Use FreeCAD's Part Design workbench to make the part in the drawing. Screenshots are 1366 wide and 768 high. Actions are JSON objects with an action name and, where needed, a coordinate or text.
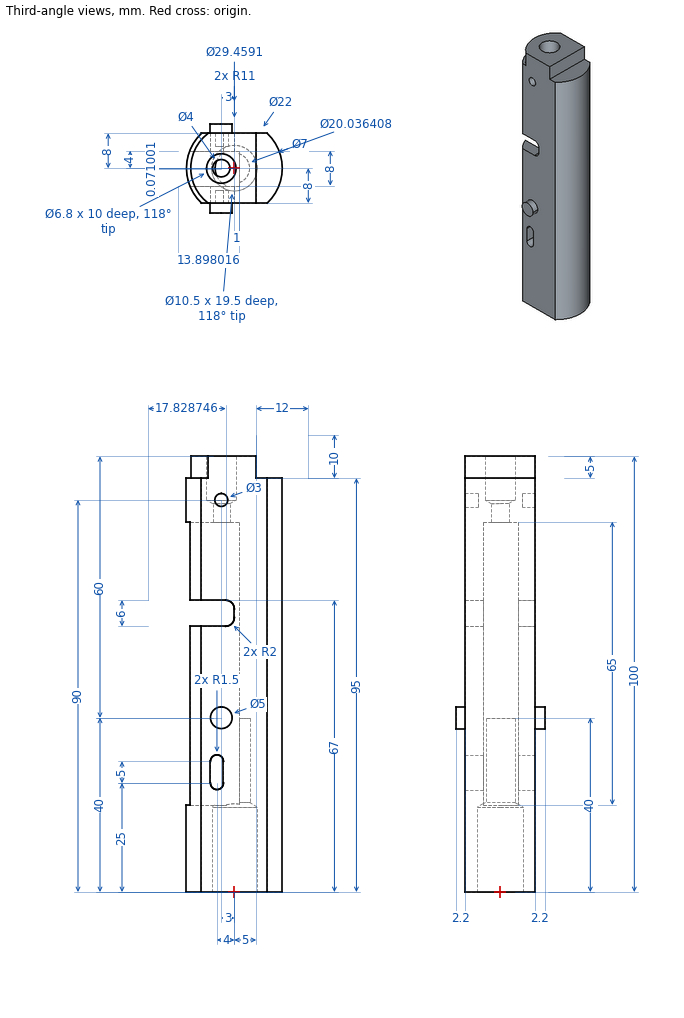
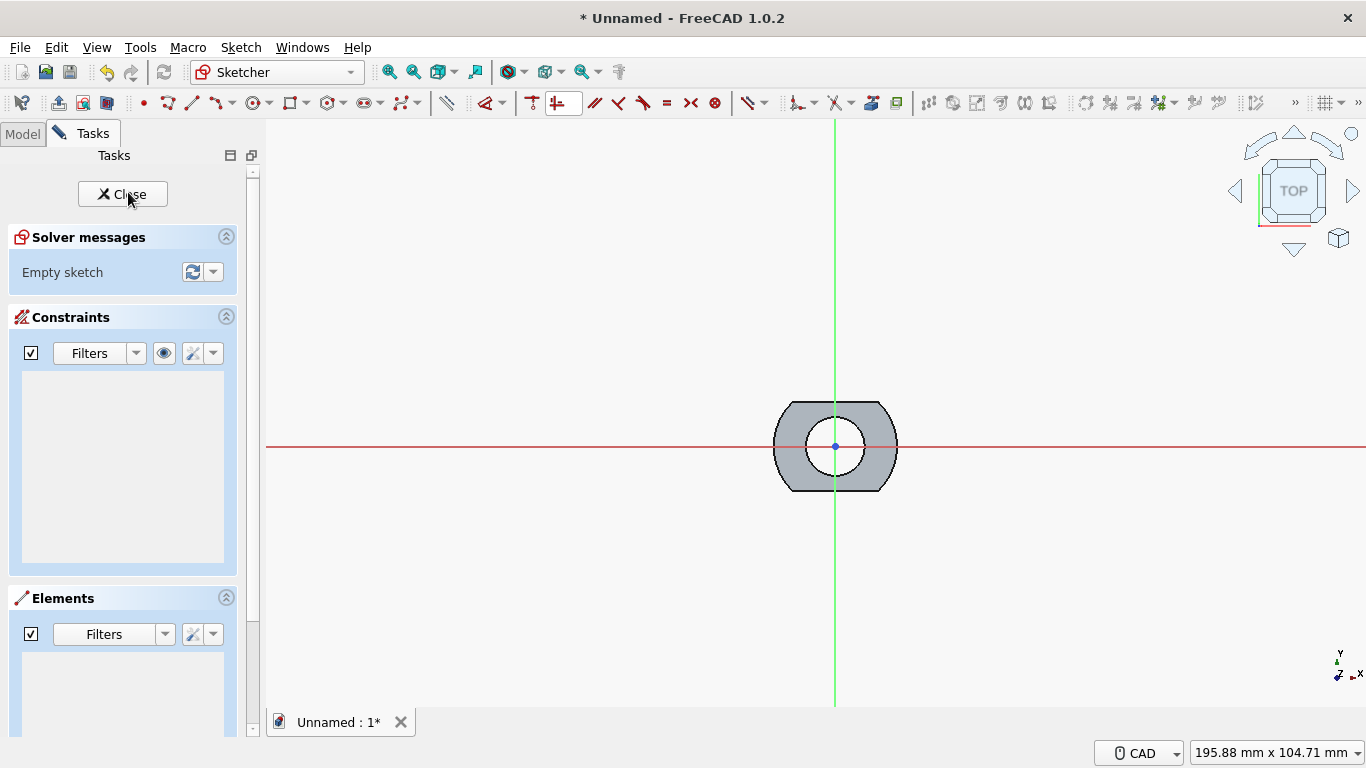
{"action": "scroll", "coordinate": [846, 451], "scroll_direction": "up", "scroll_amount": 11}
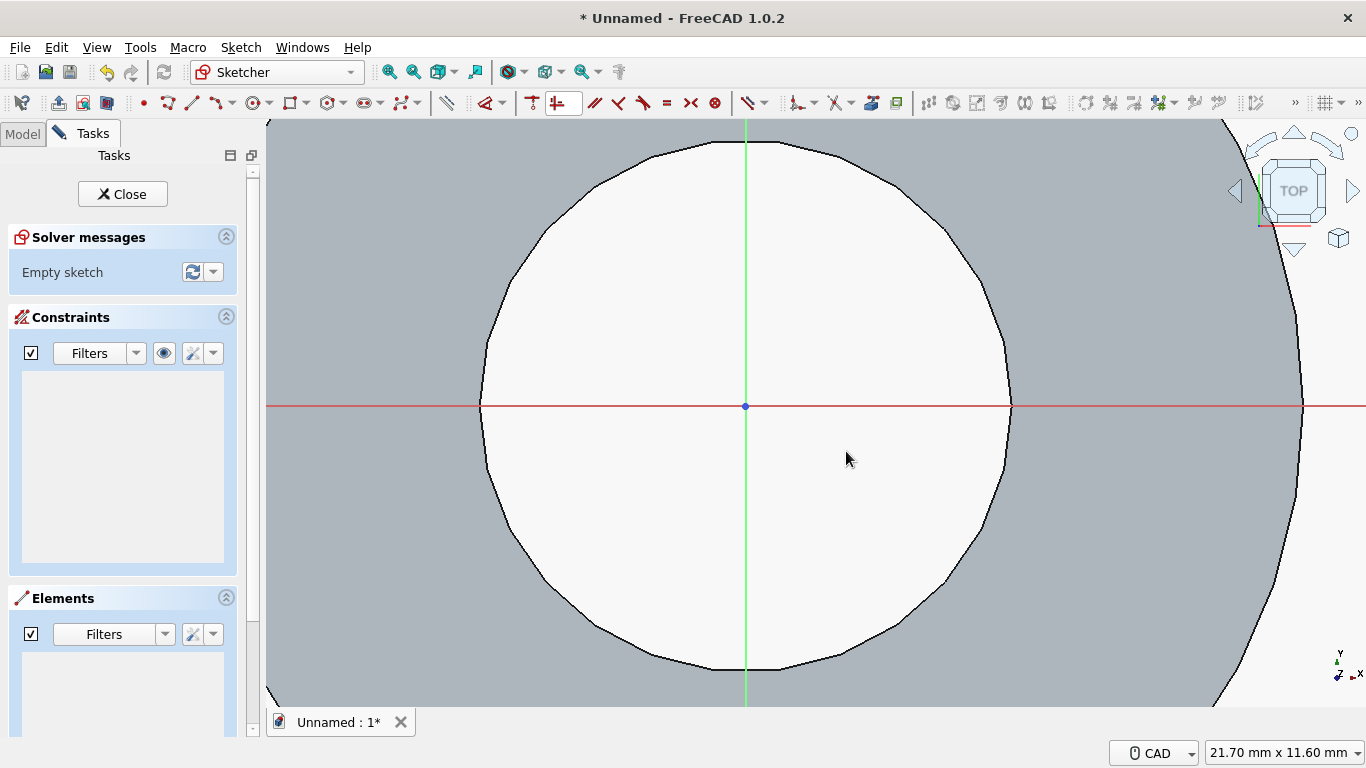
{"action": "left_click", "coordinate": [254, 104]}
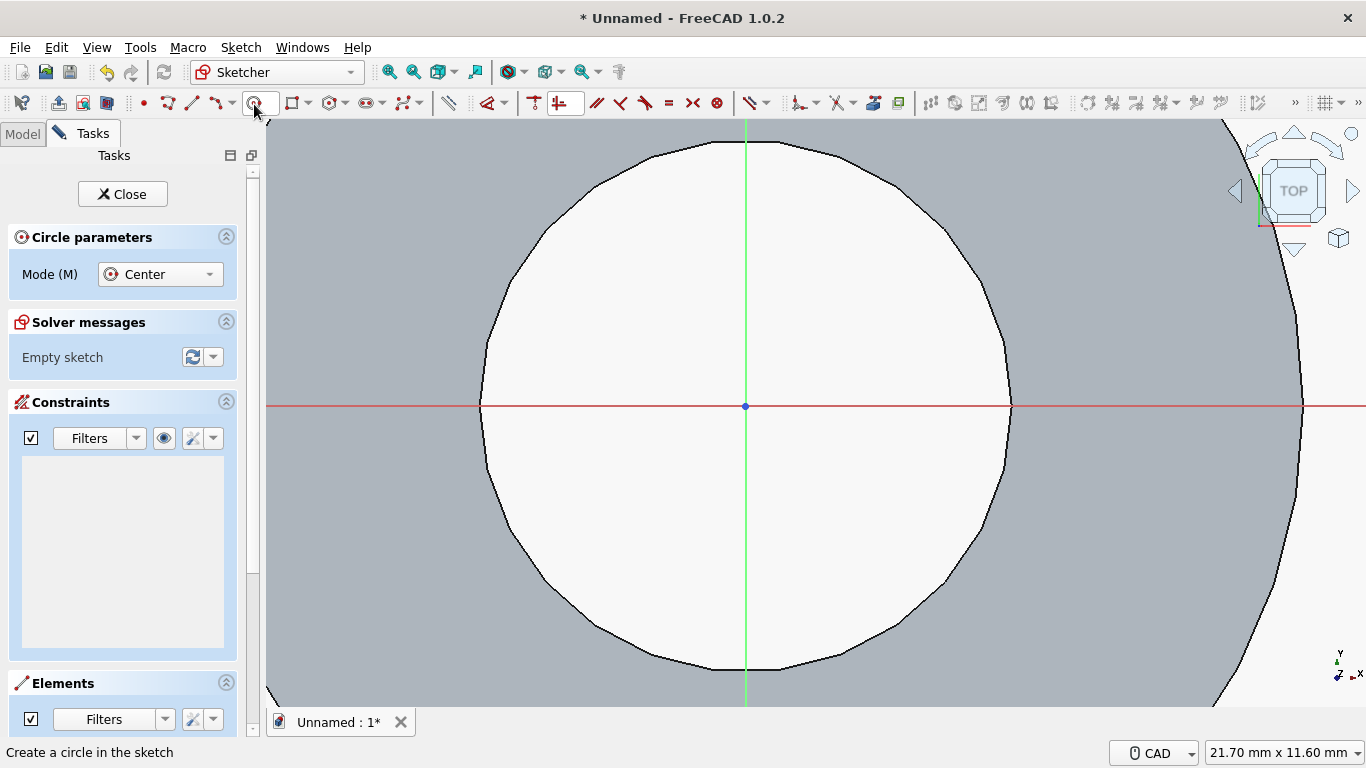
{"action": "left_click", "coordinate": [746, 406]}
{"action": "mouse_move", "coordinate": [871, 281]}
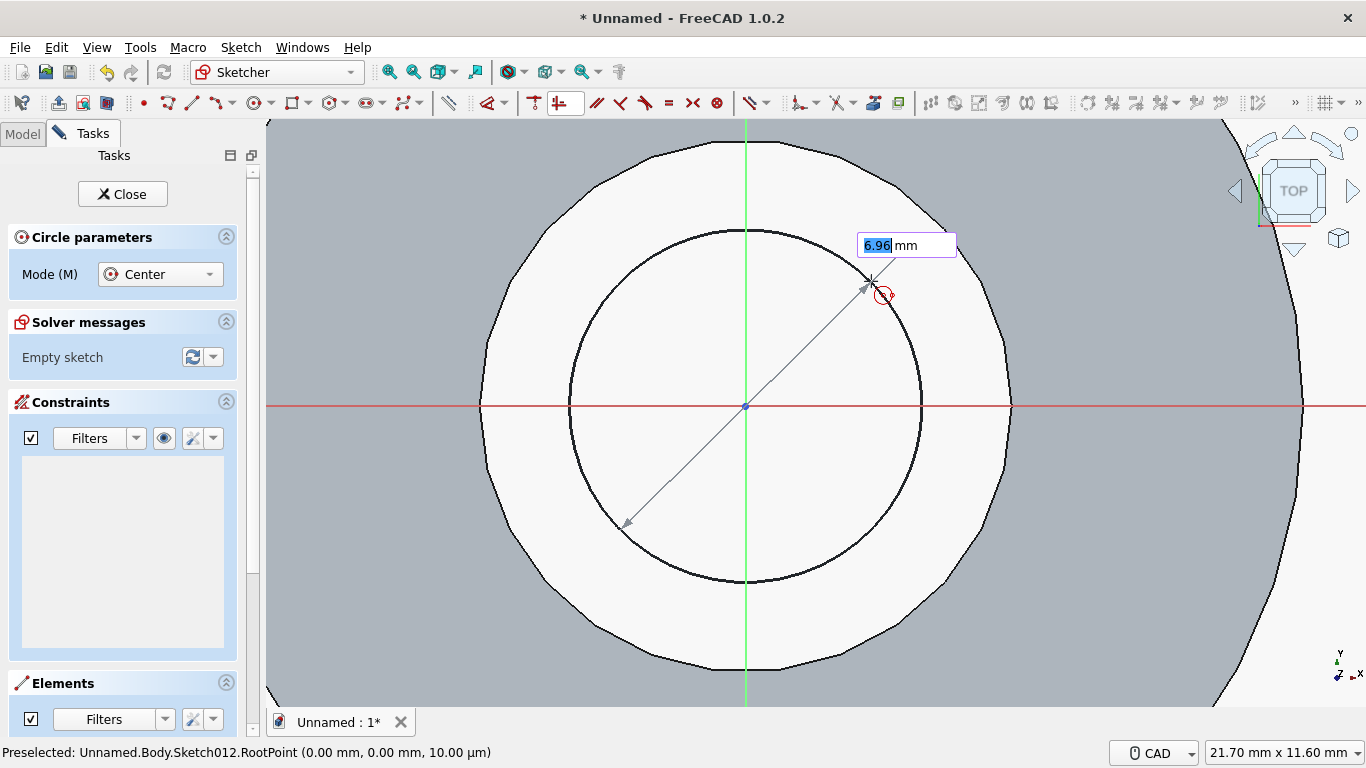
{"action": "type", "text": "7"}
{"action": "key", "text": "Return"}
{"action": "key", "text": "Escape"}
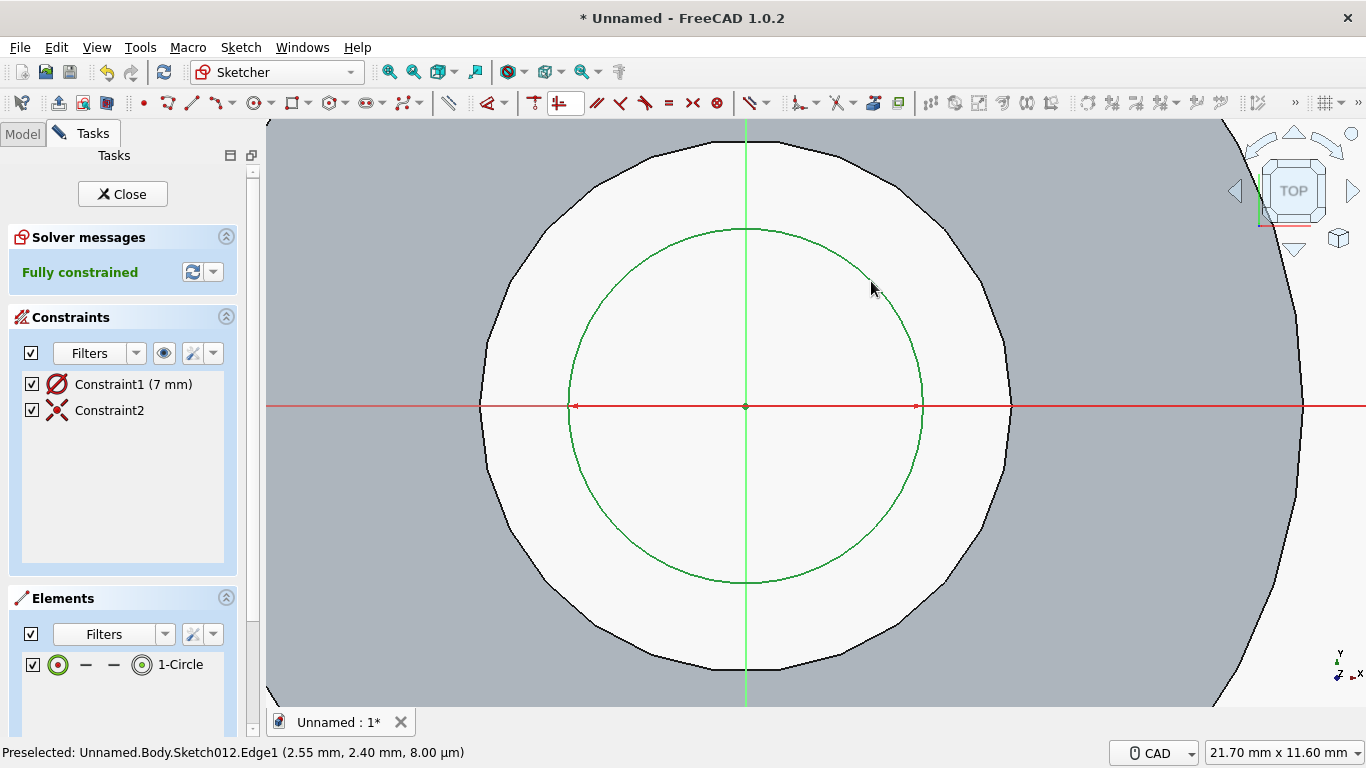
{"action": "left_click", "coordinate": [123, 194]}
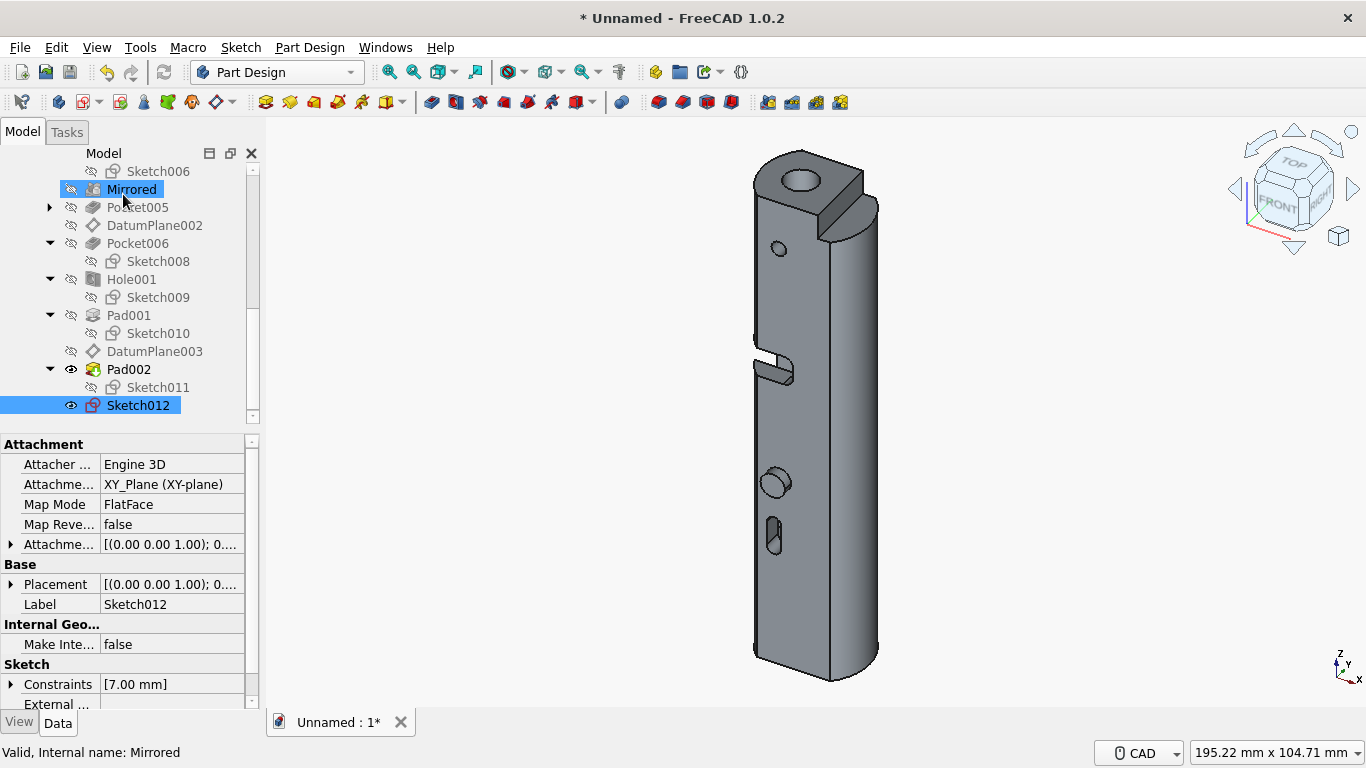
{"action": "left_click", "coordinate": [432, 102]}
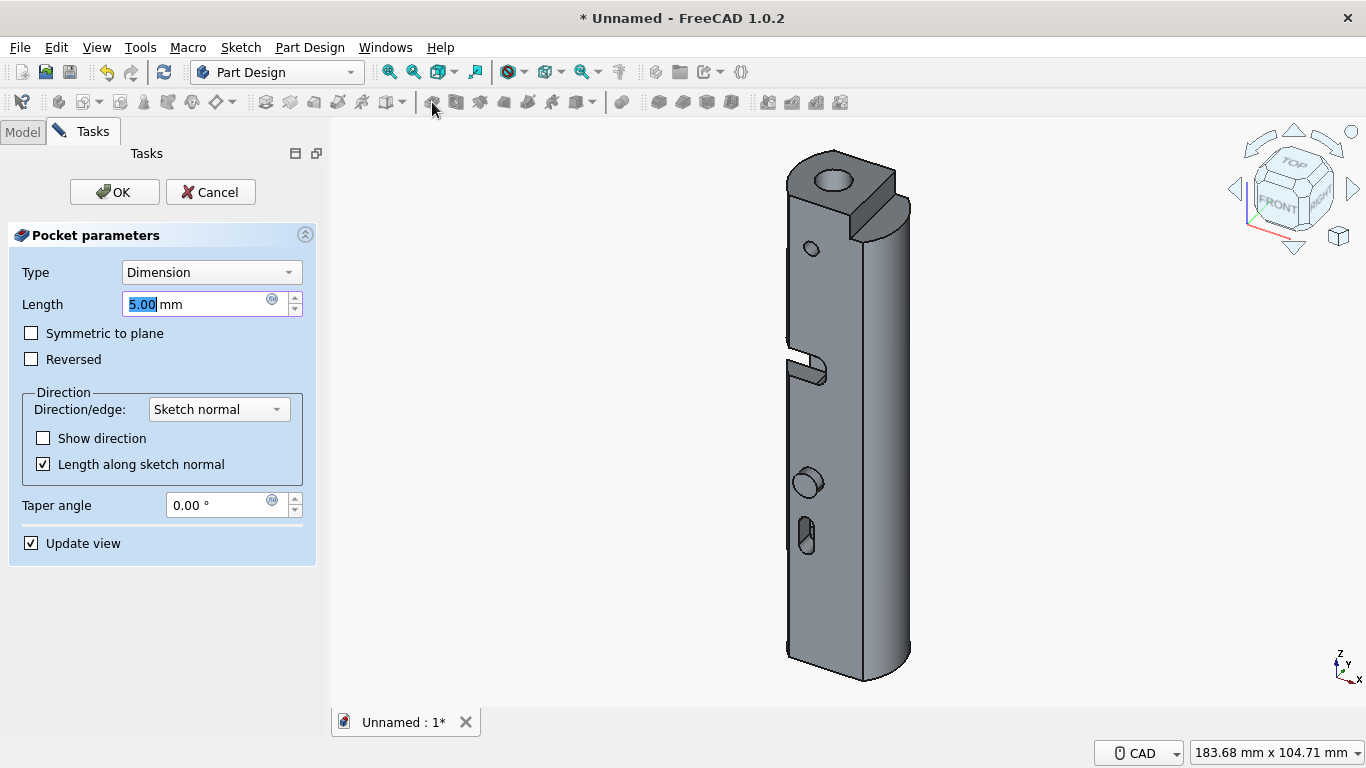
{"action": "type", "text": "40"}
{"action": "key", "text": "Tab"}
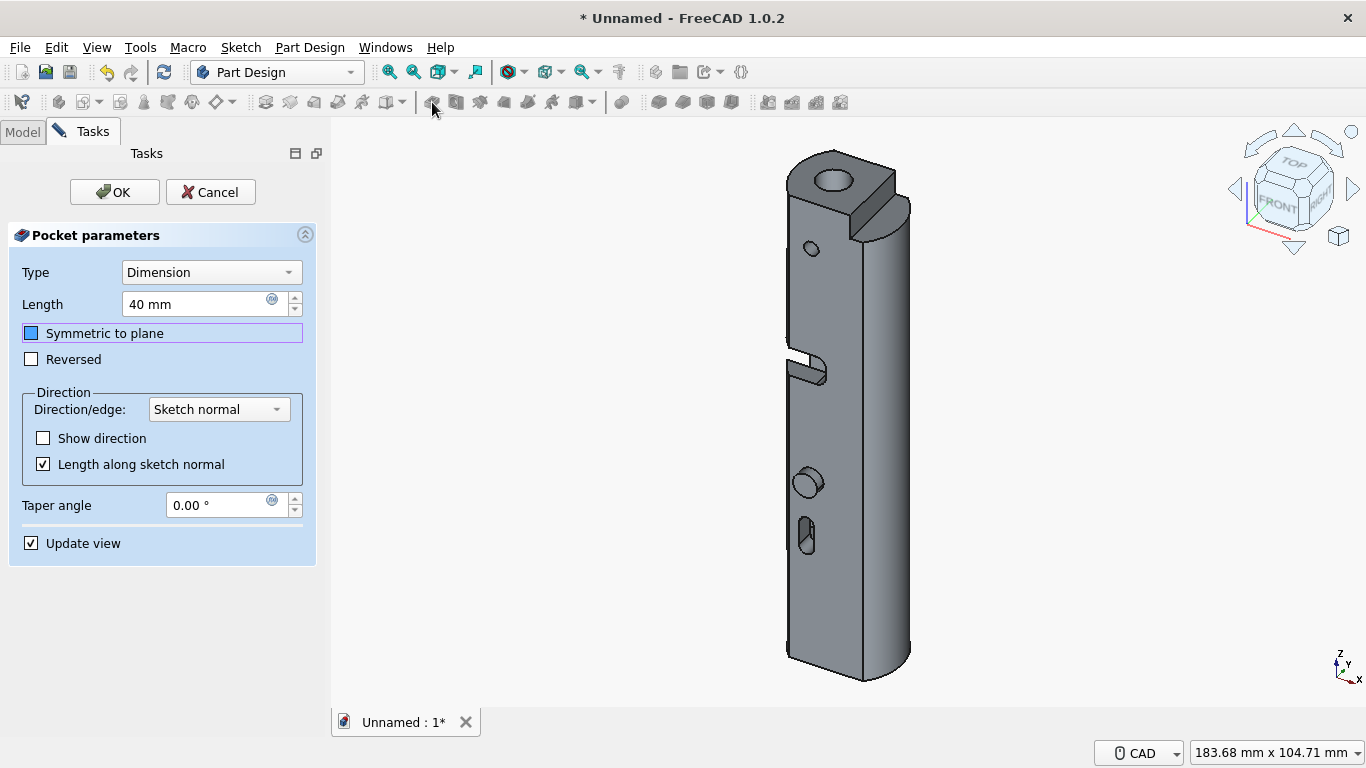
{"action": "left_click", "coordinate": [30, 359]}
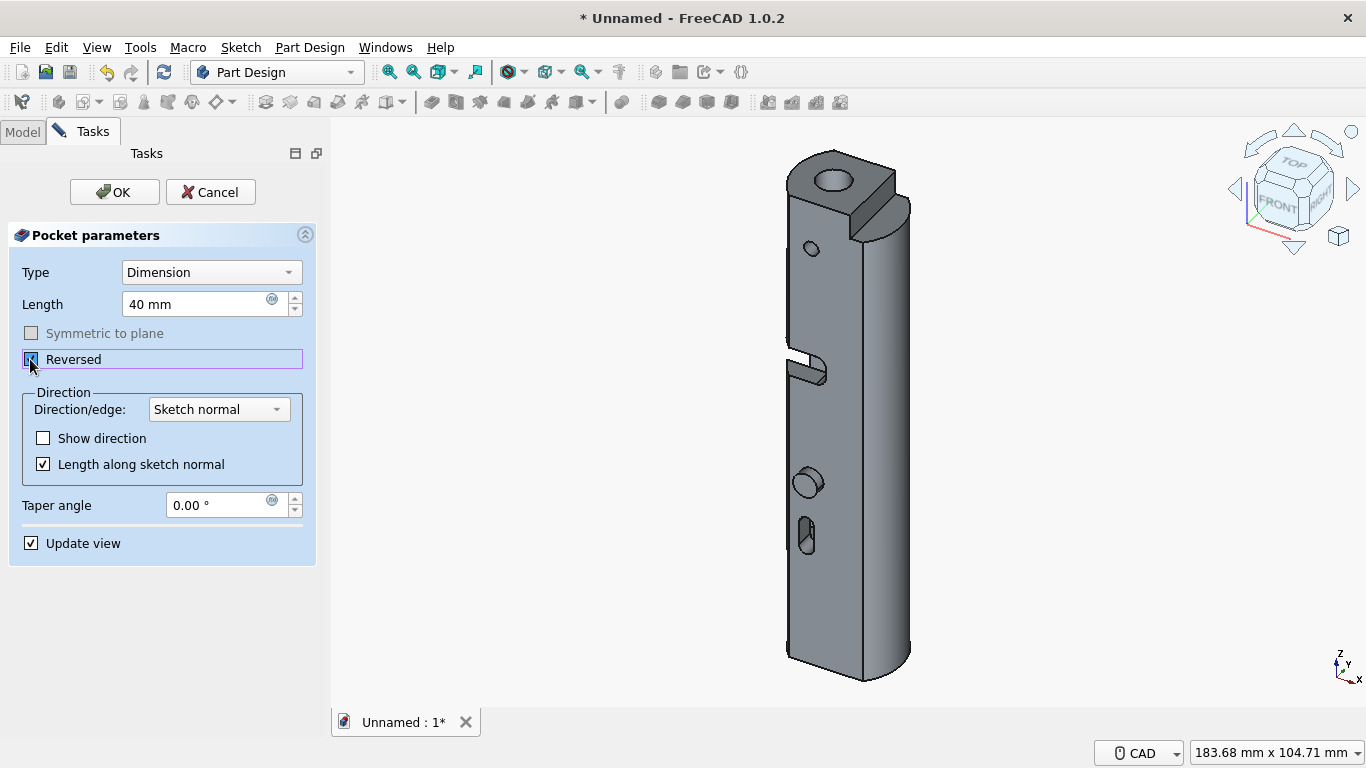
{"action": "left_click", "coordinate": [115, 192]}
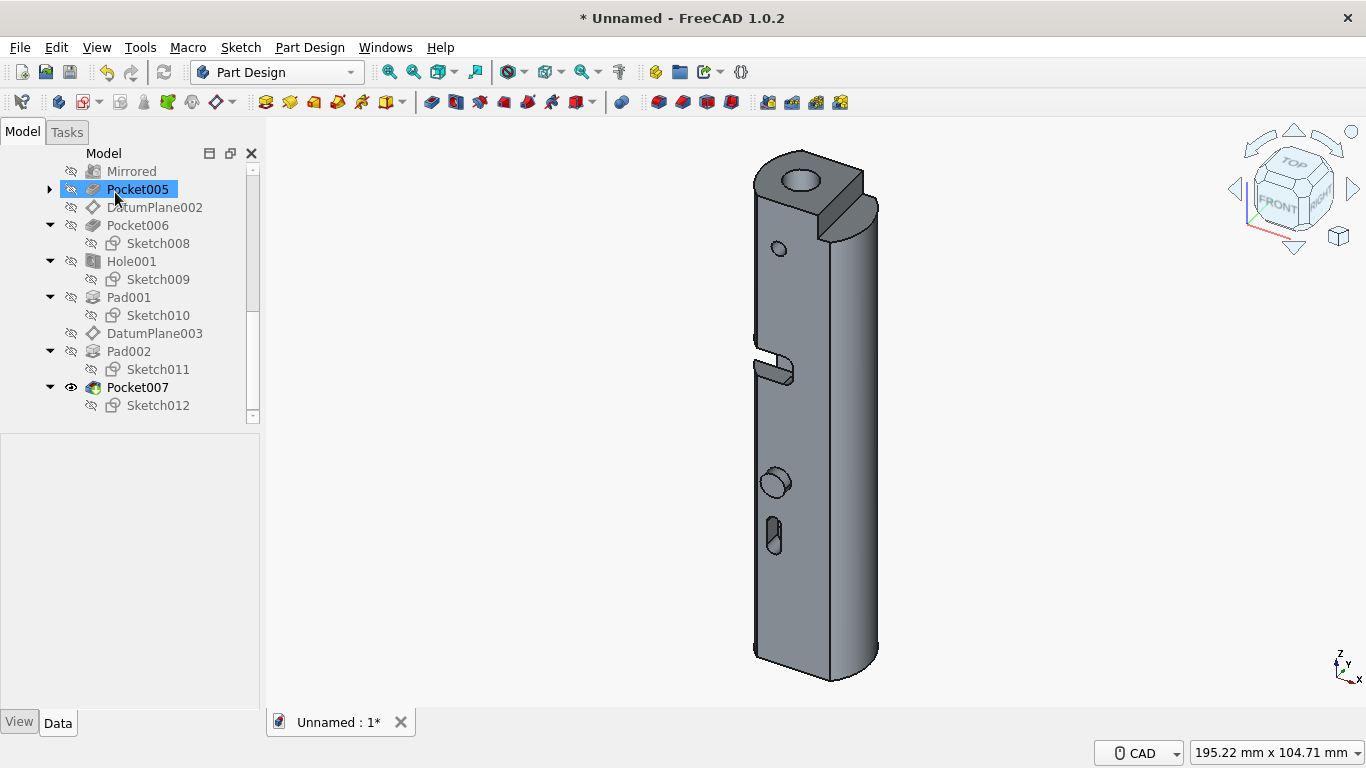
{"action": "left_click", "coordinate": [837, 174]}